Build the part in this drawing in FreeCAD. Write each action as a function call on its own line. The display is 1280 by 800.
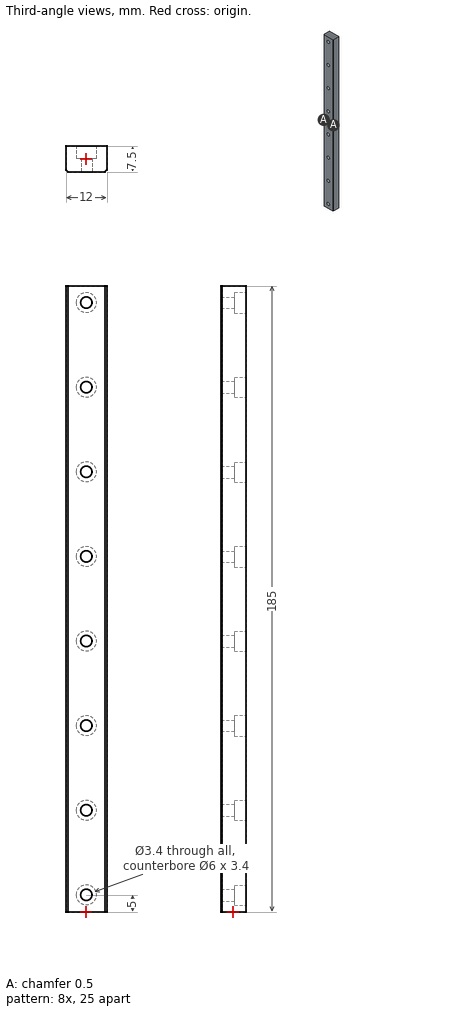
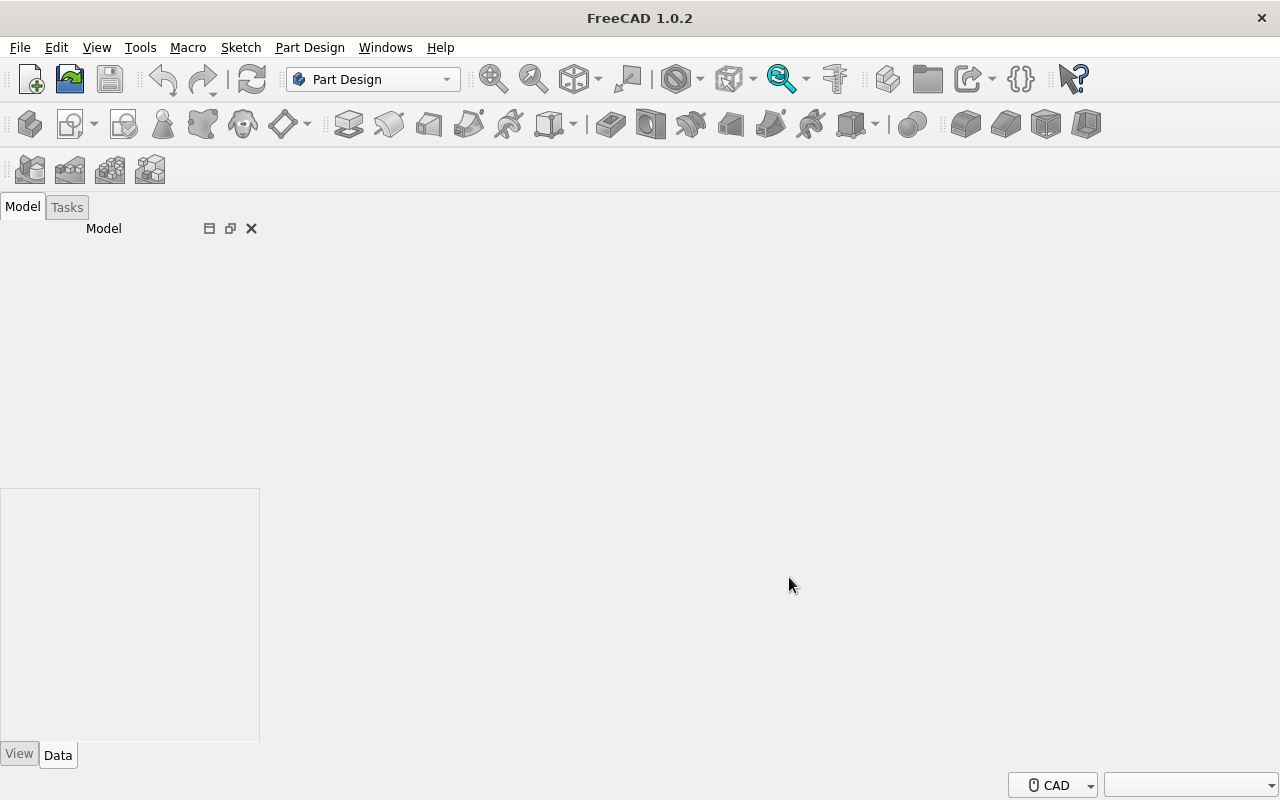
click(30, 80)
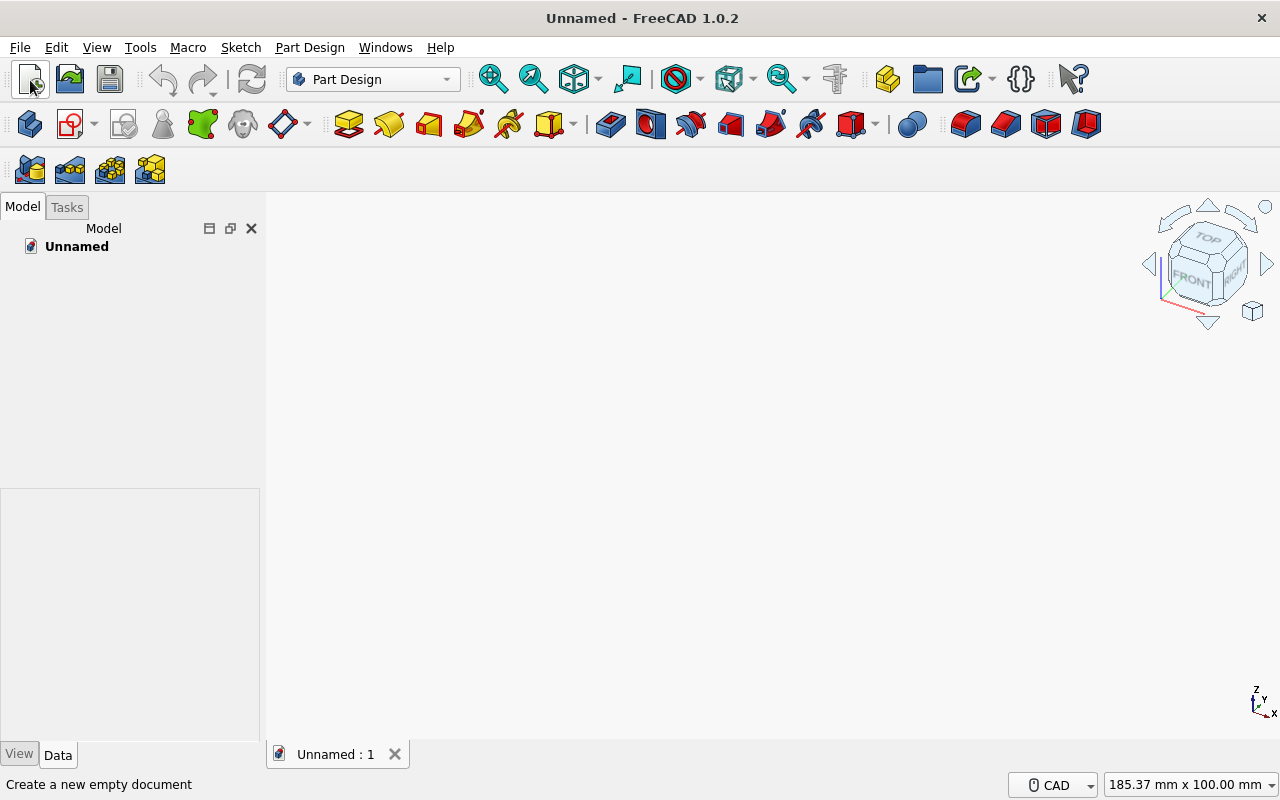
click(70, 124)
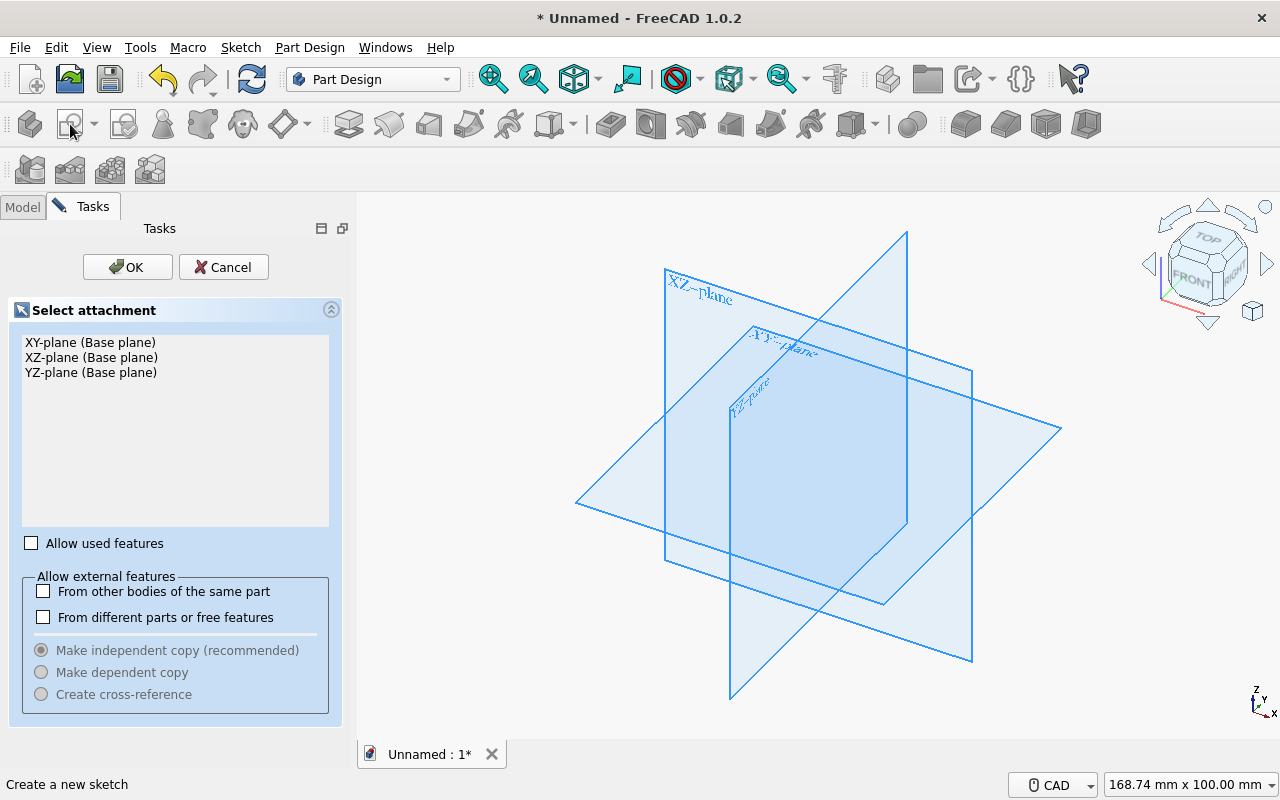
click(82, 342)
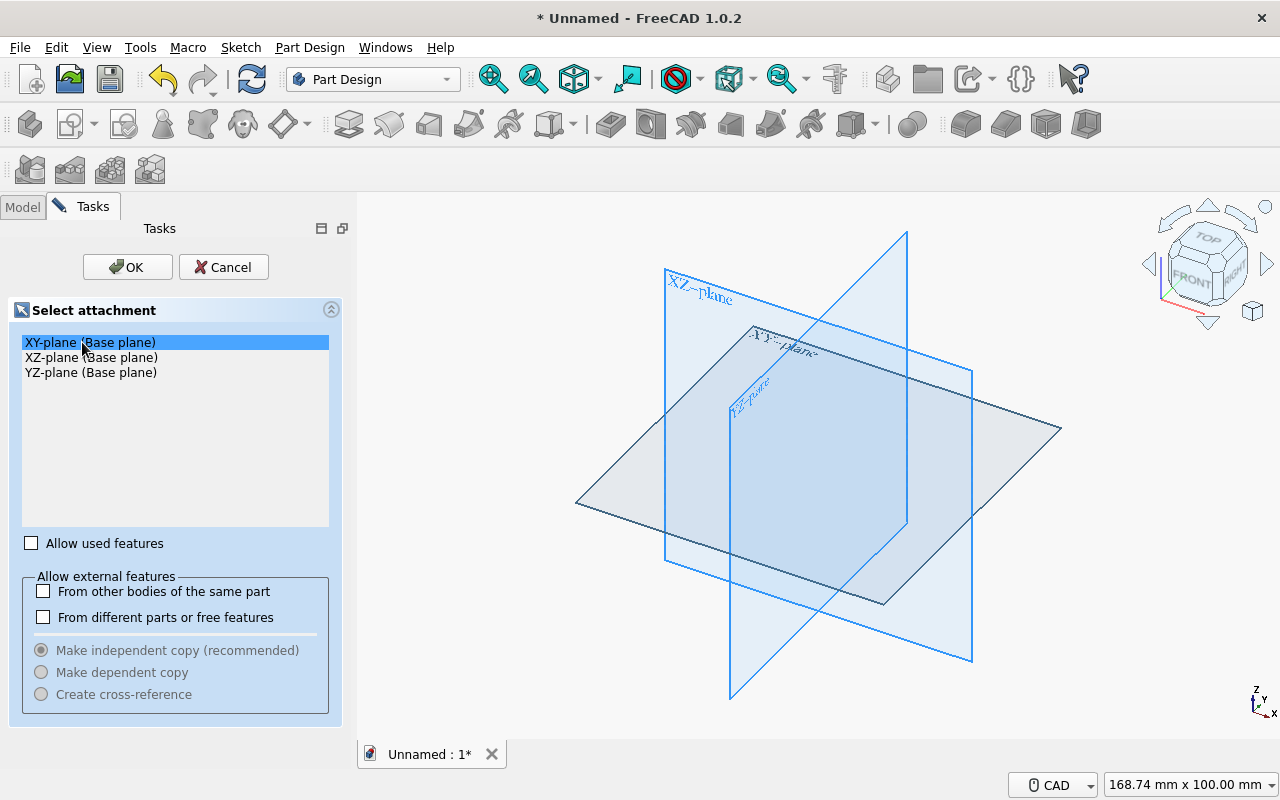
click(128, 267)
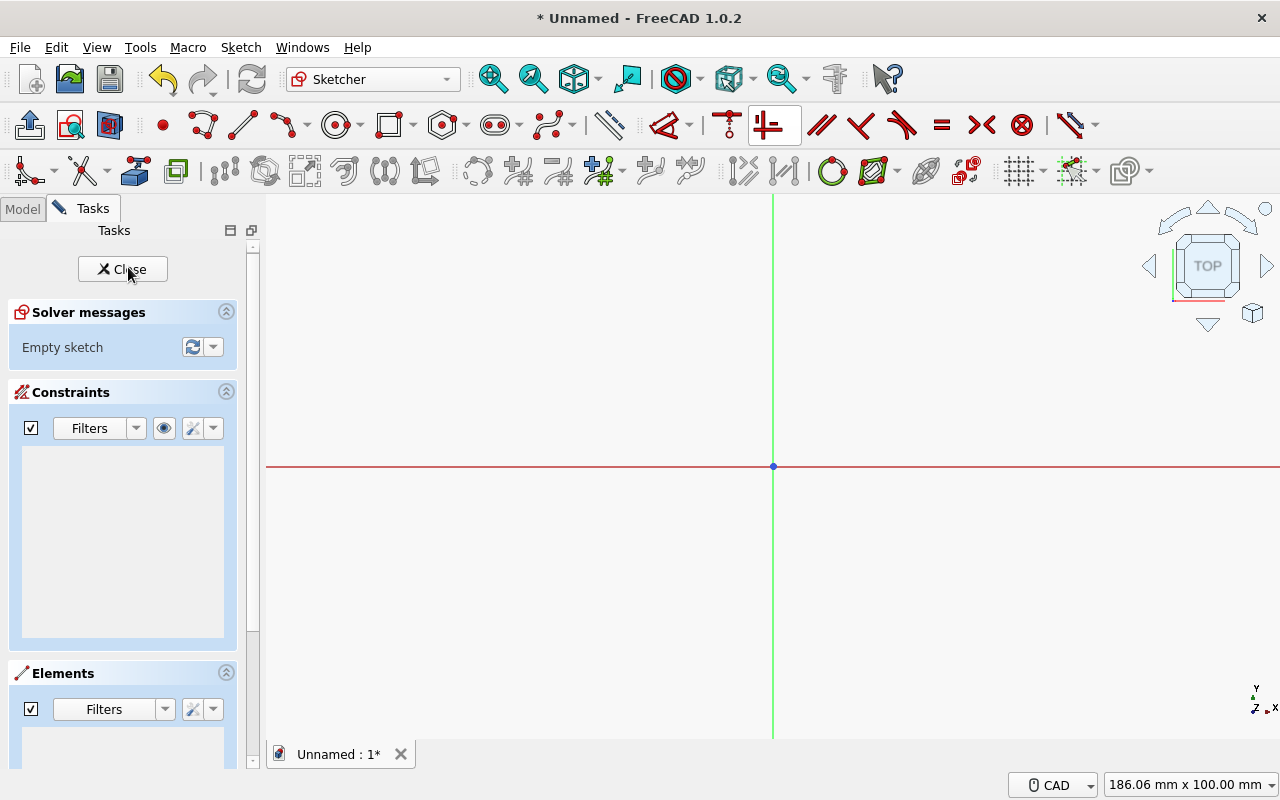
scroll(782, 466, up, 11)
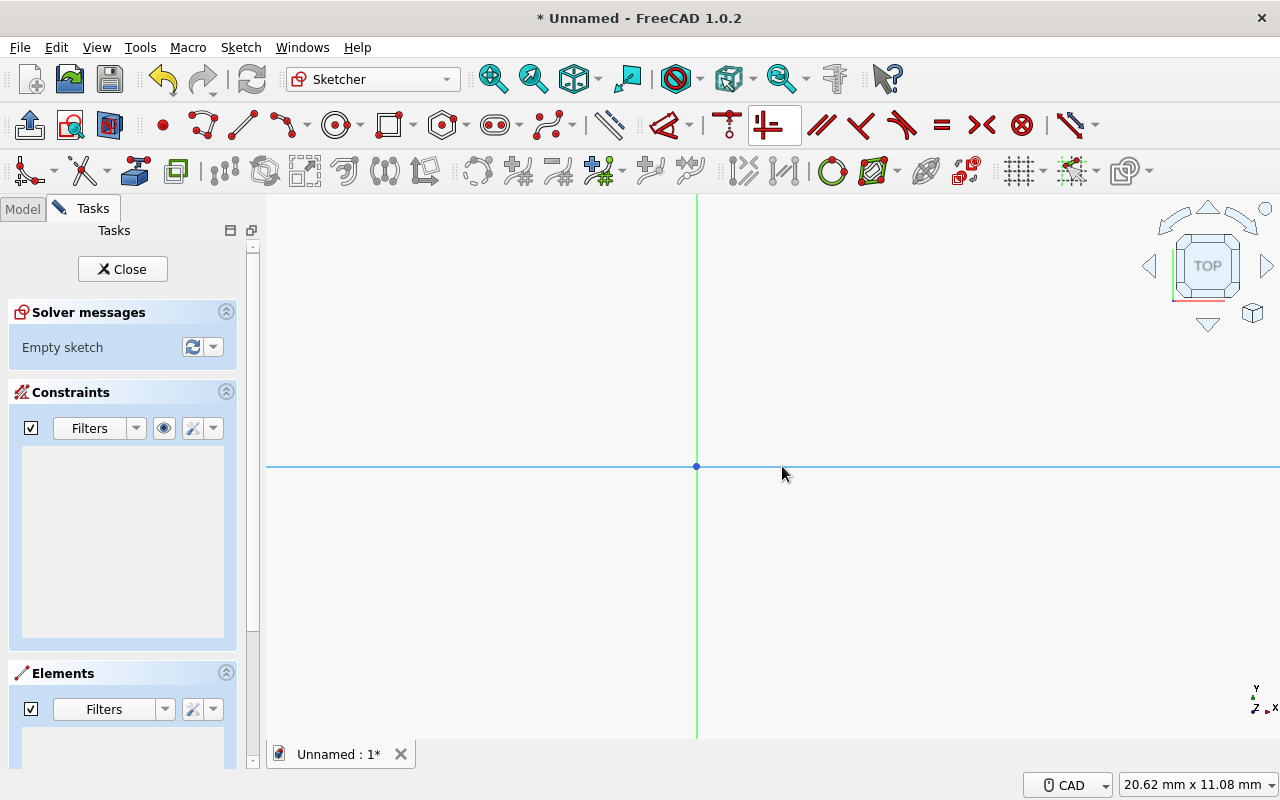
click(416, 126)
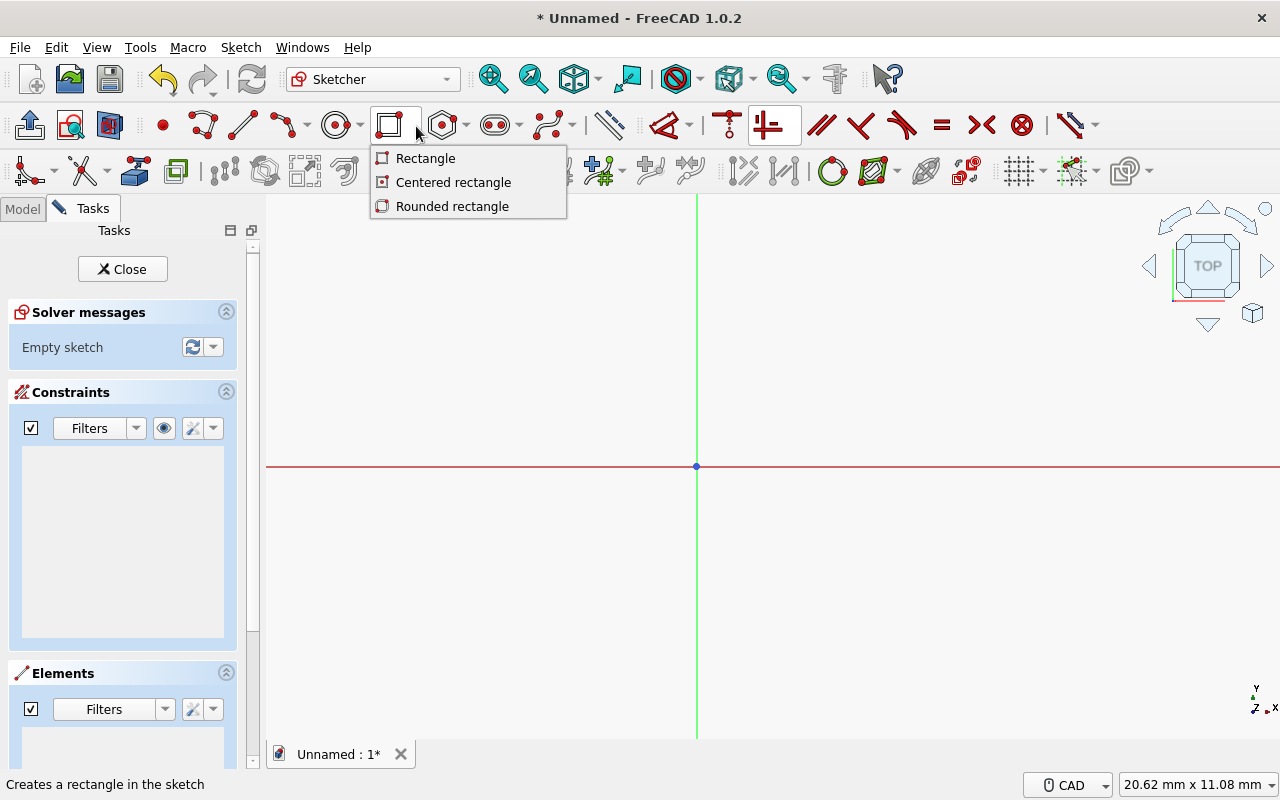
click(468, 182)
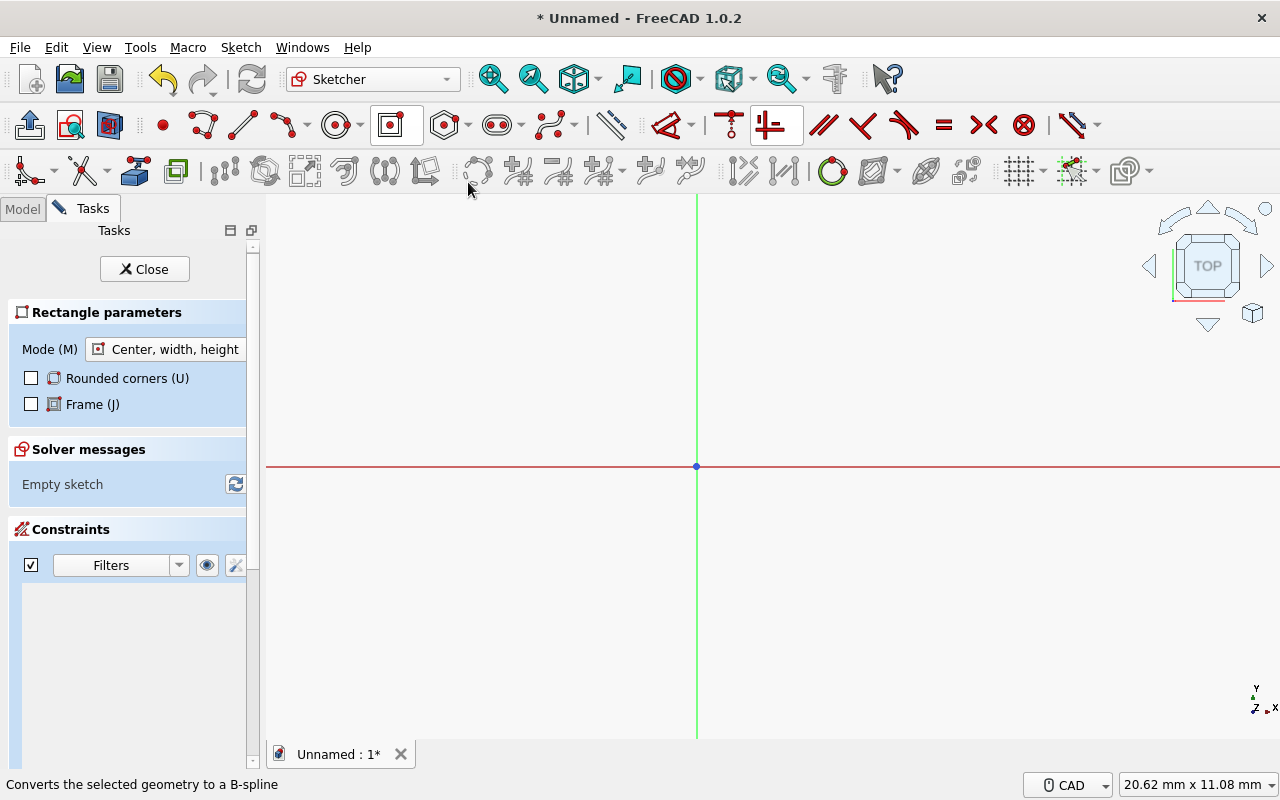
click(697, 466)
click(992, 282)
key(Escape)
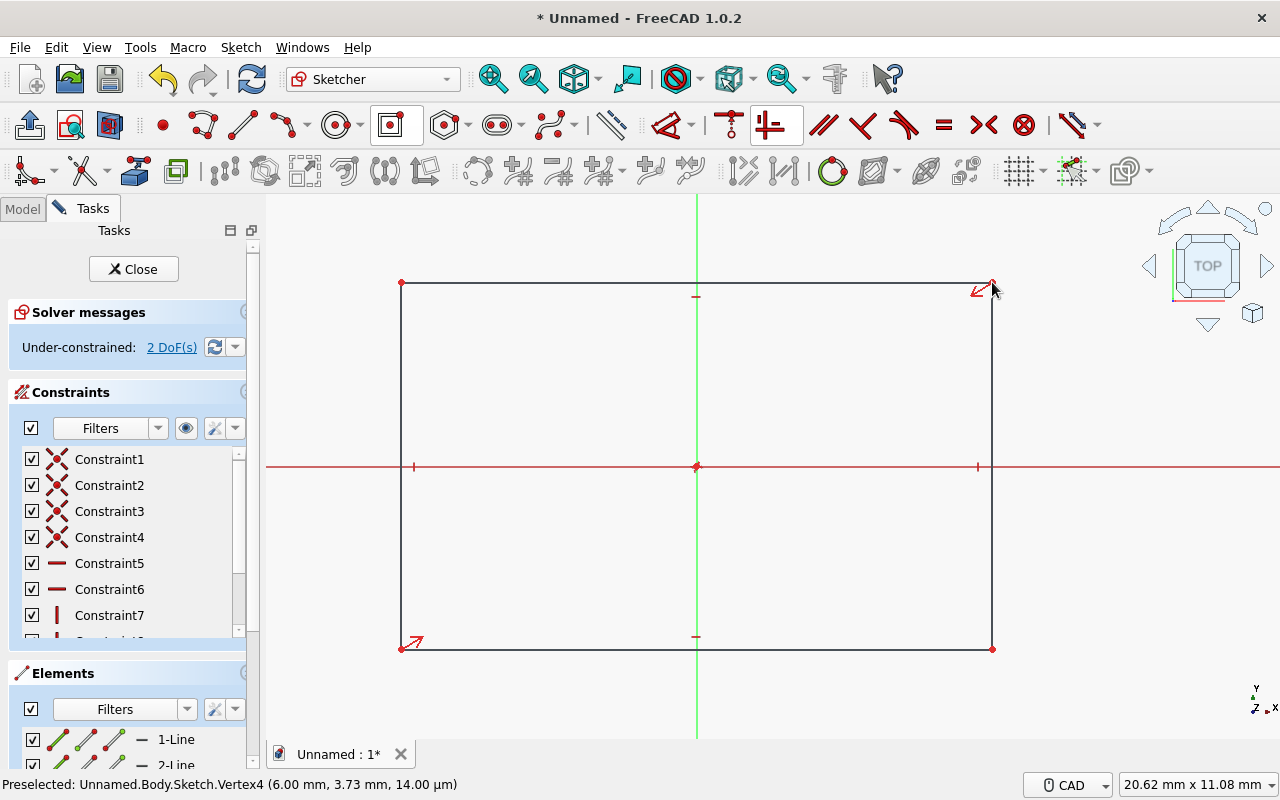
click(579, 650)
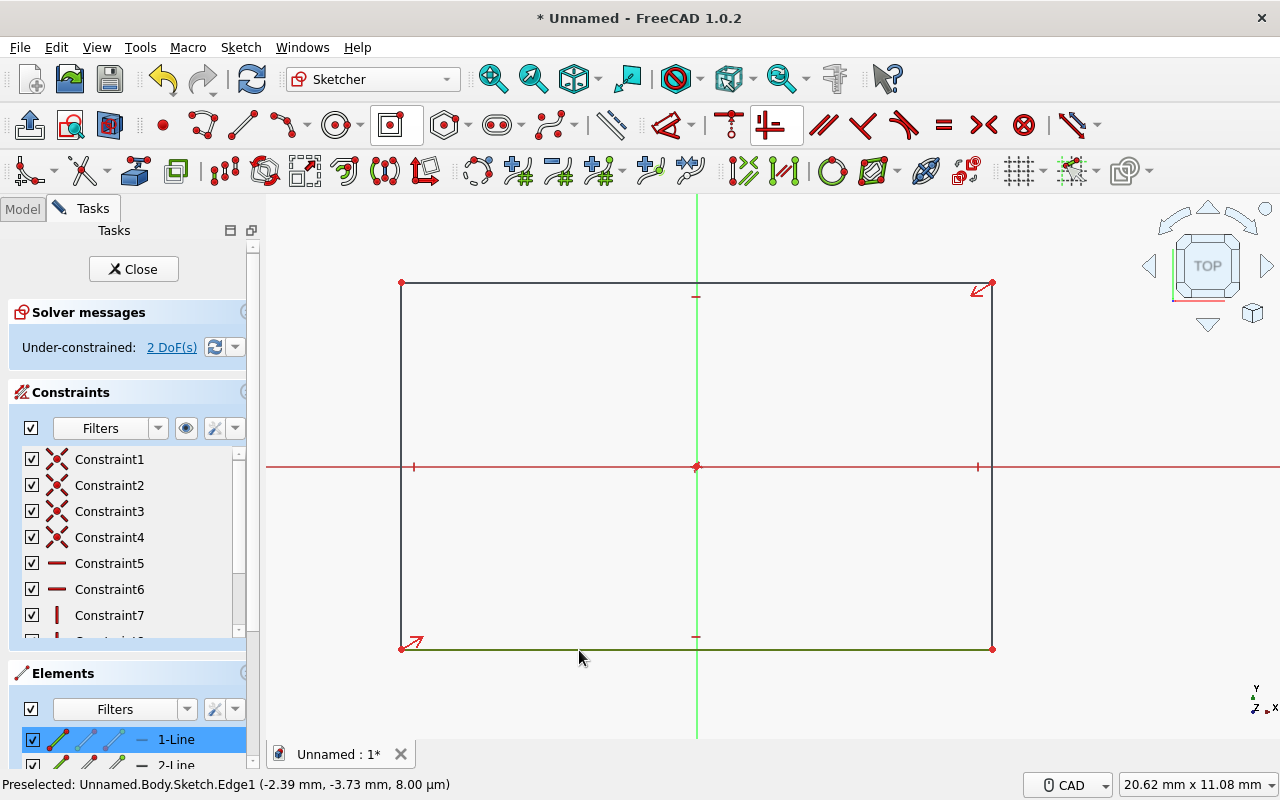
key(l)